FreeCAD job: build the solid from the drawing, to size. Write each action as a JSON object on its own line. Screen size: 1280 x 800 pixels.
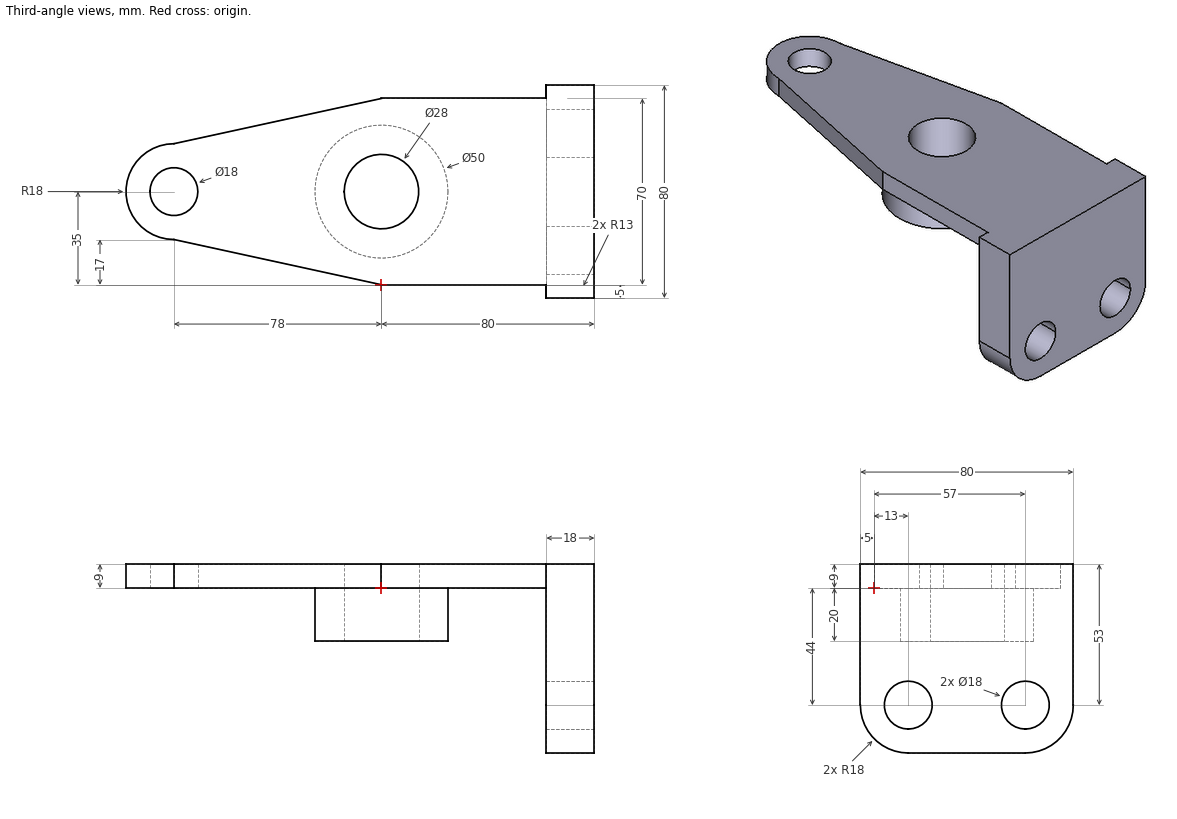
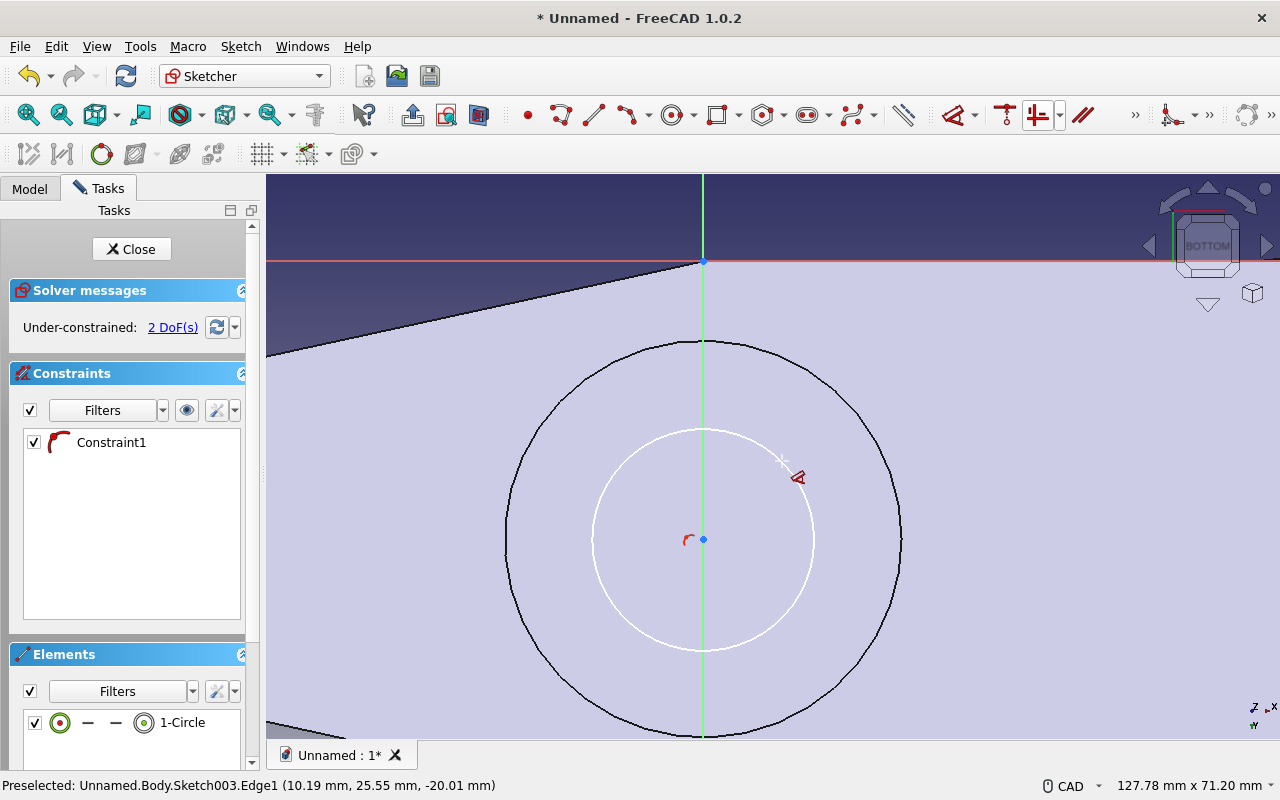
{"action": "left_click", "coordinate": [781, 461]}
{"action": "left_click", "coordinate": [803, 438]}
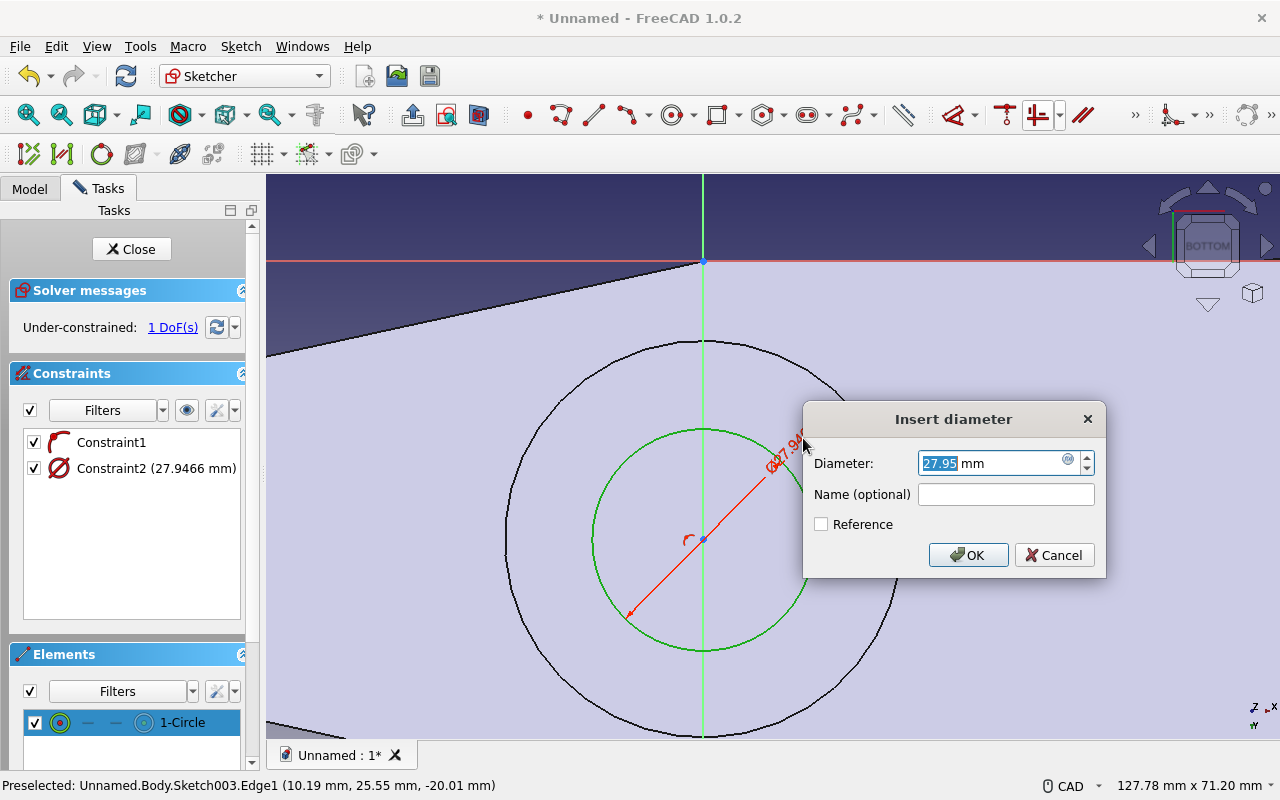
{"action": "type", "text": "28"}
{"action": "key", "text": "Return"}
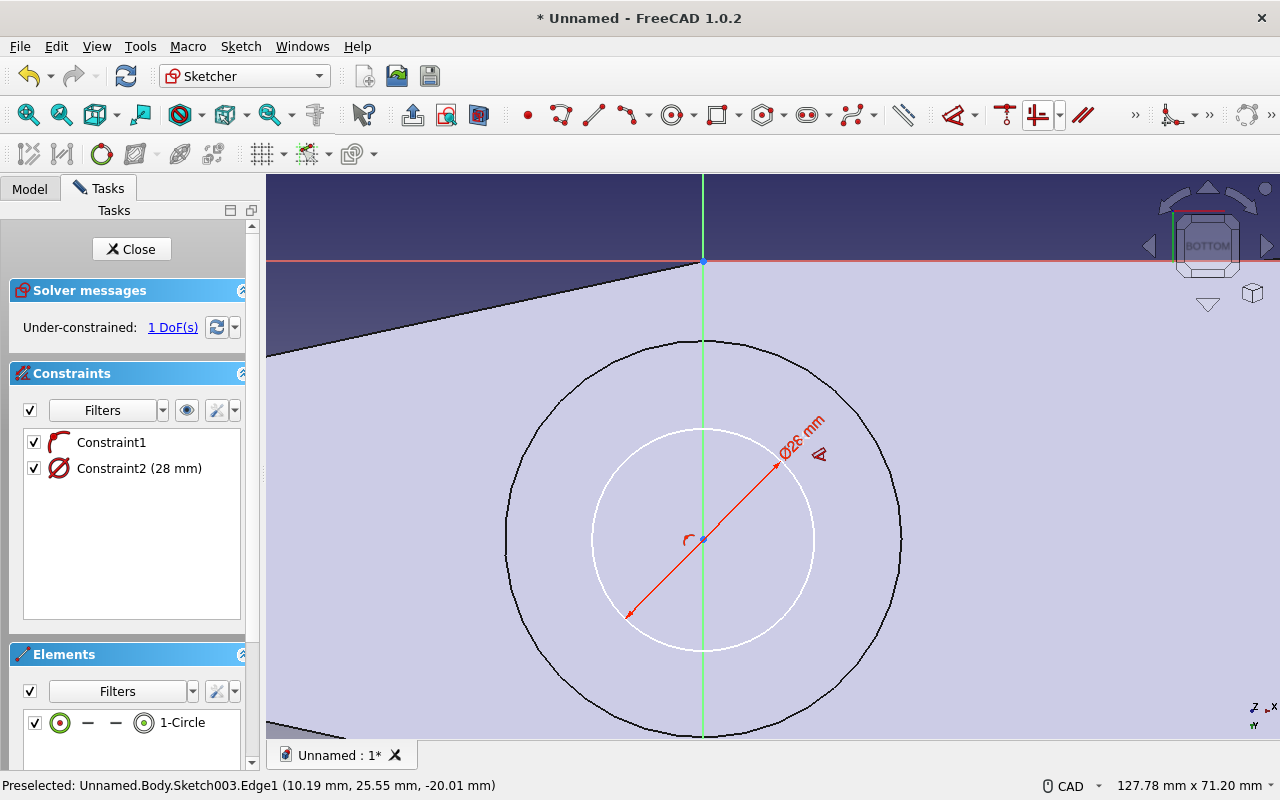
{"action": "left_click", "coordinate": [703, 540]}
{"action": "left_click", "coordinate": [737, 401]}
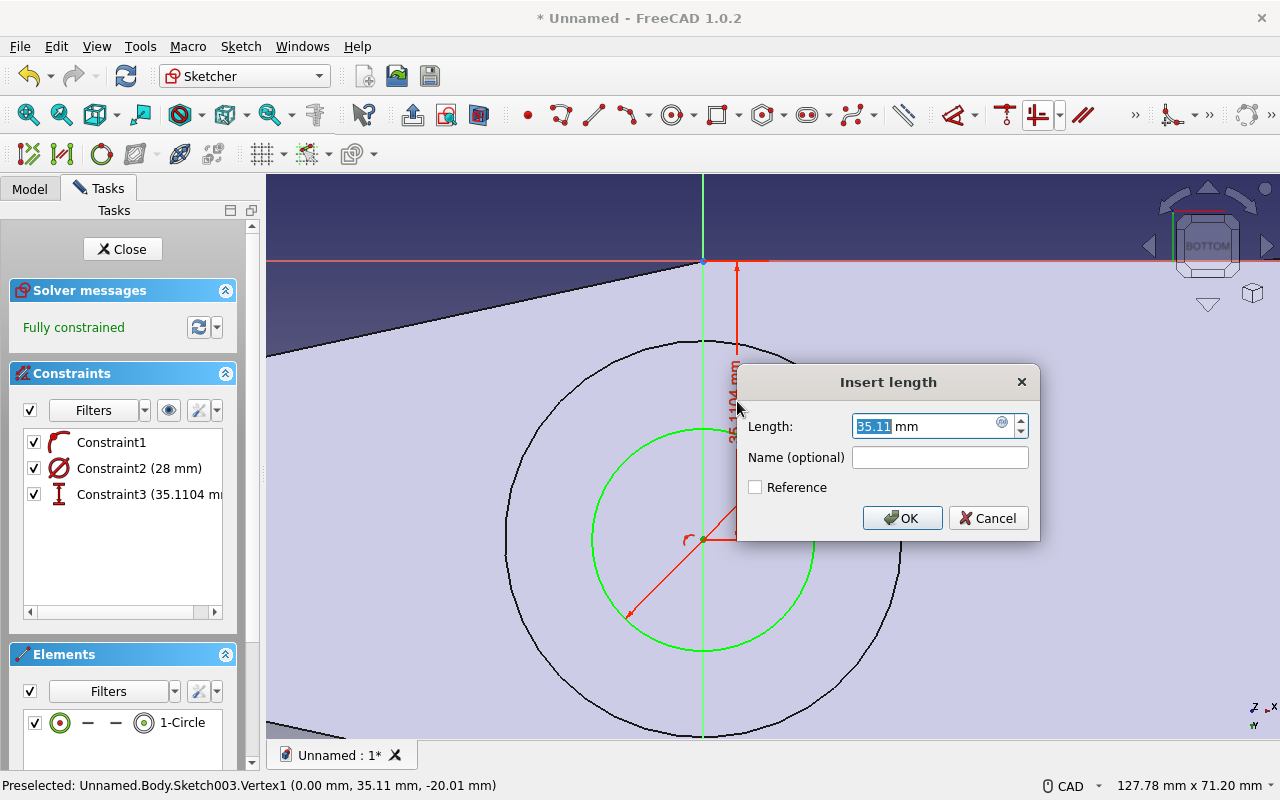
{"action": "type", "text": "35"}
{"action": "key", "text": "Return"}
{"action": "key", "text": "Escape"}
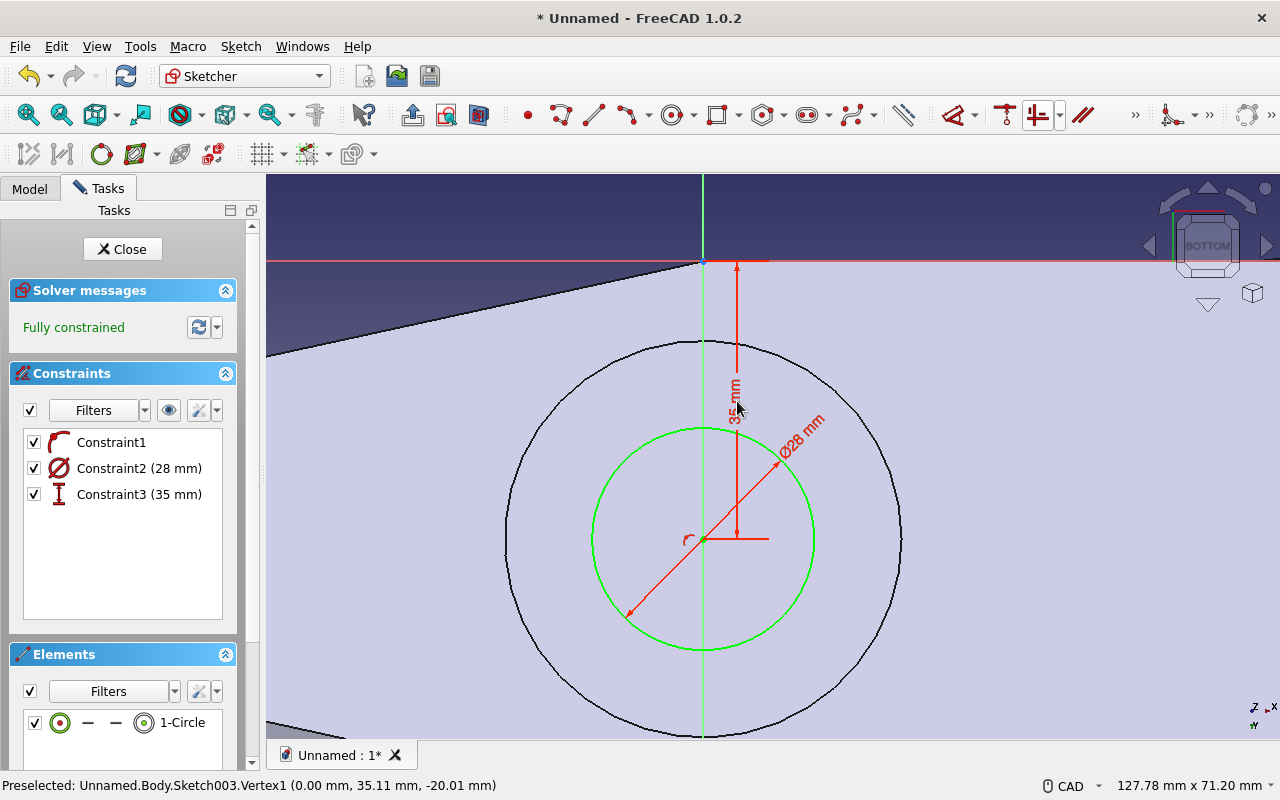
{"action": "left_click", "coordinate": [123, 249]}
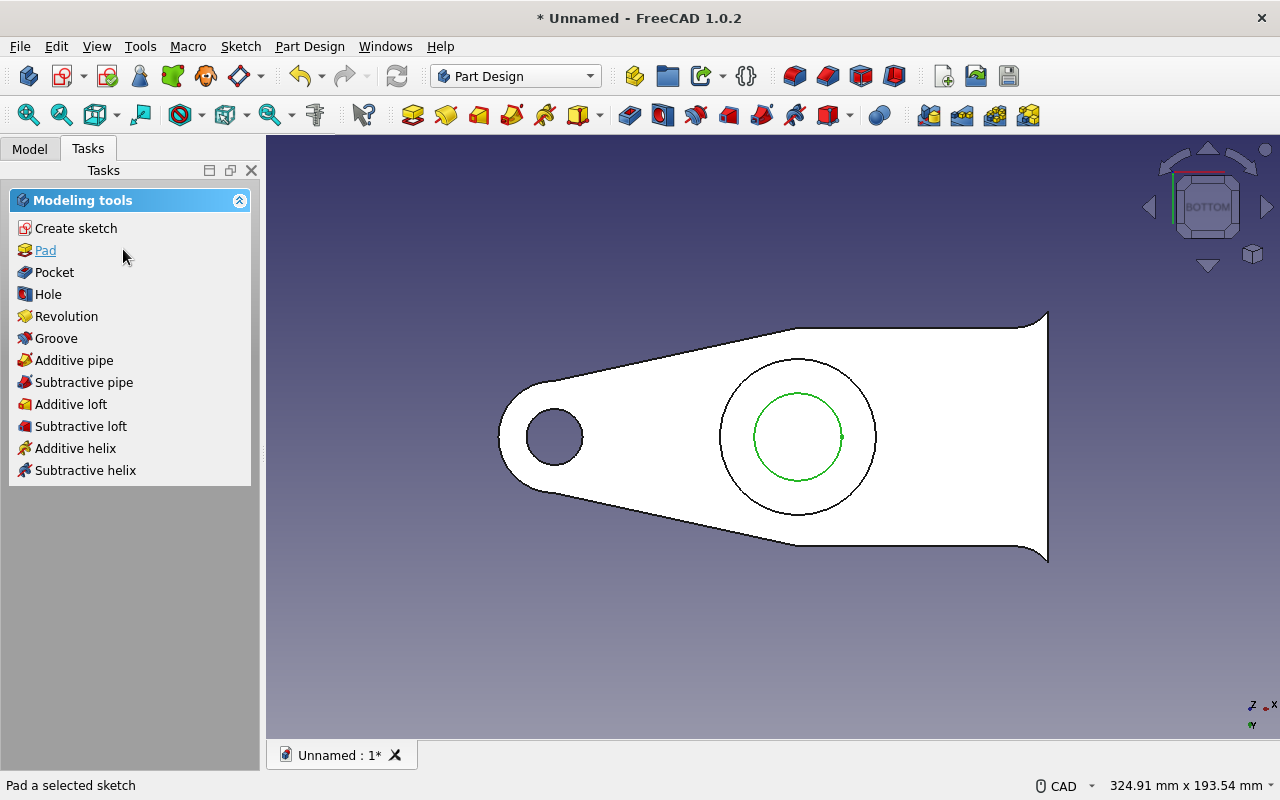
{"action": "left_click", "coordinate": [630, 116]}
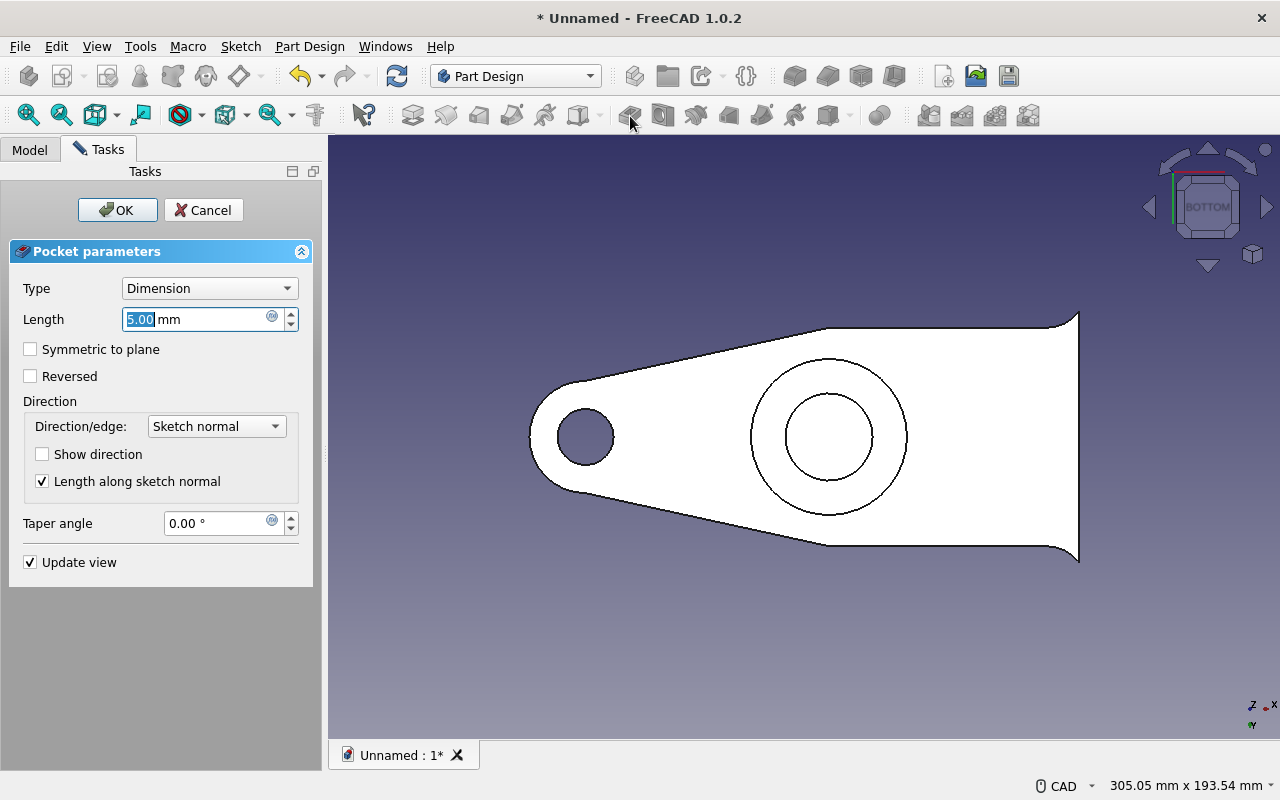
{"action": "left_click", "coordinate": [210, 288]}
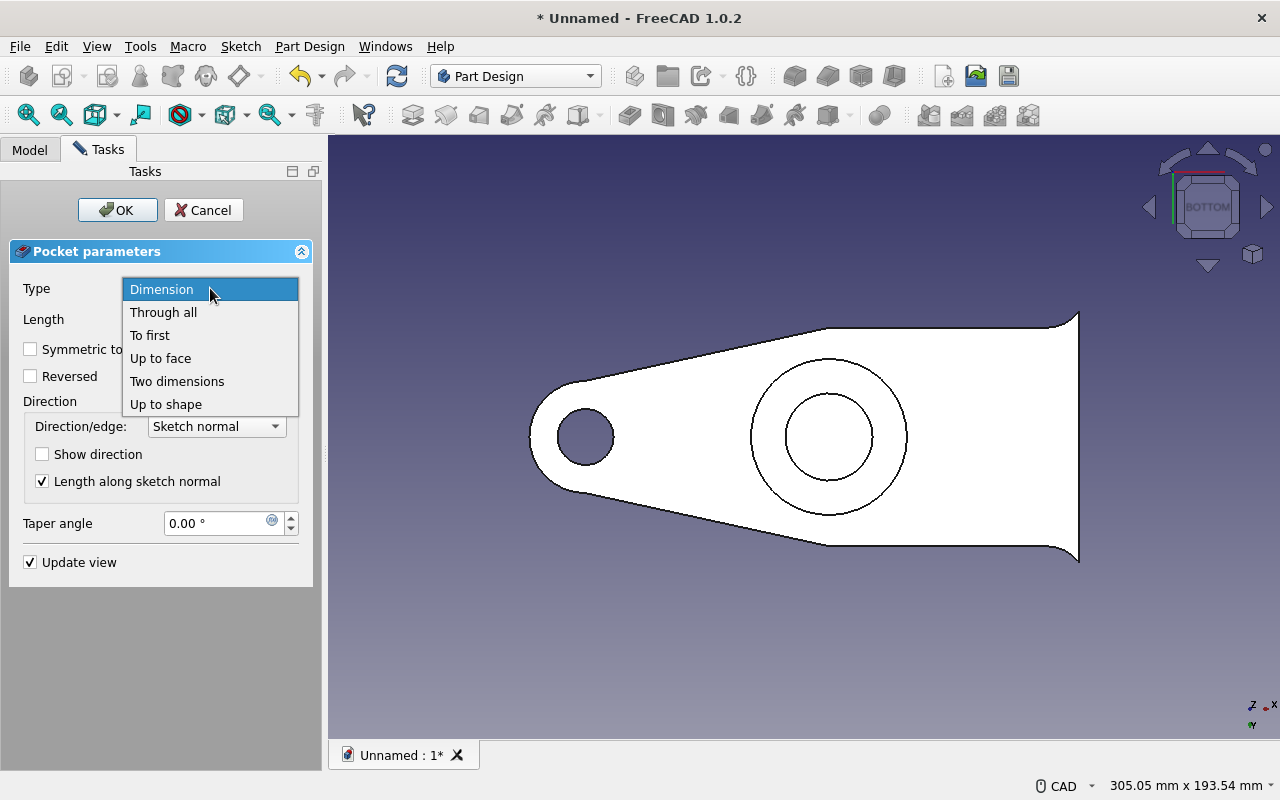
{"action": "left_click", "coordinate": [208, 312]}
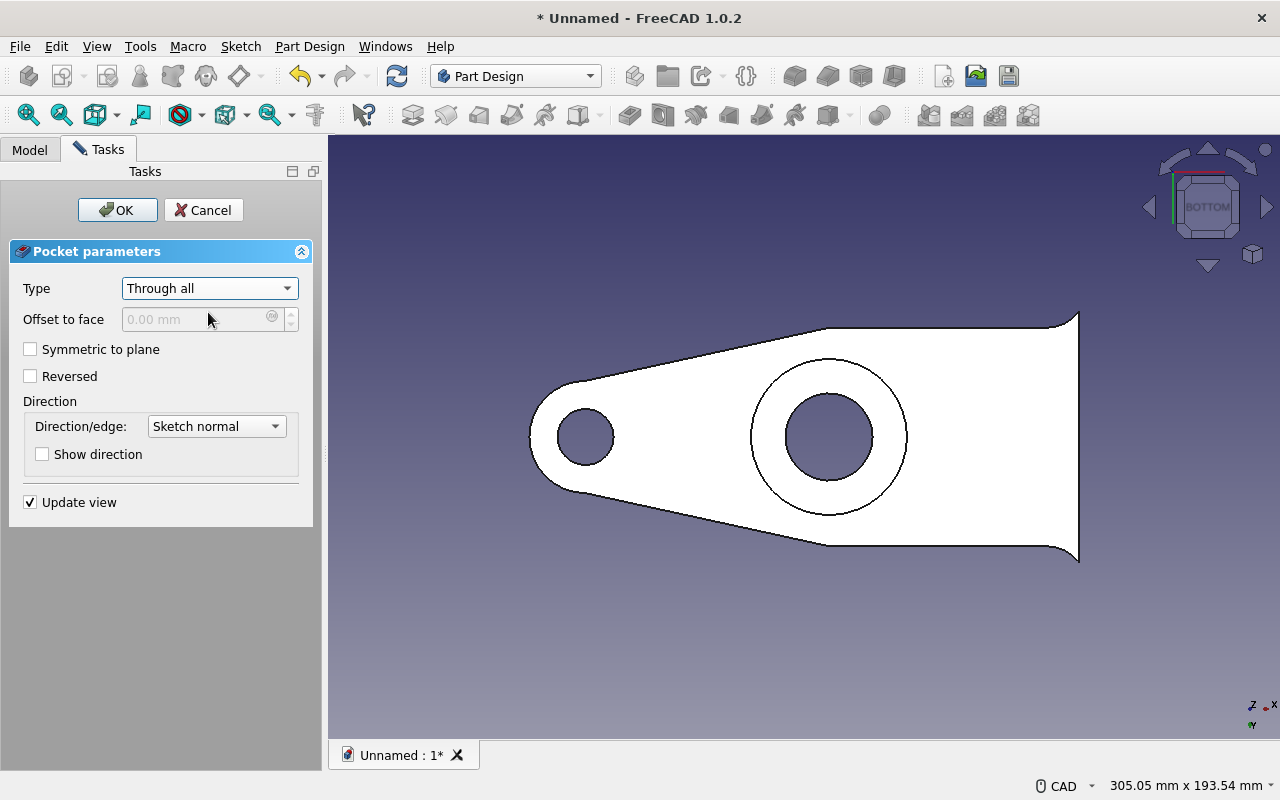
{"action": "left_click", "coordinate": [118, 210]}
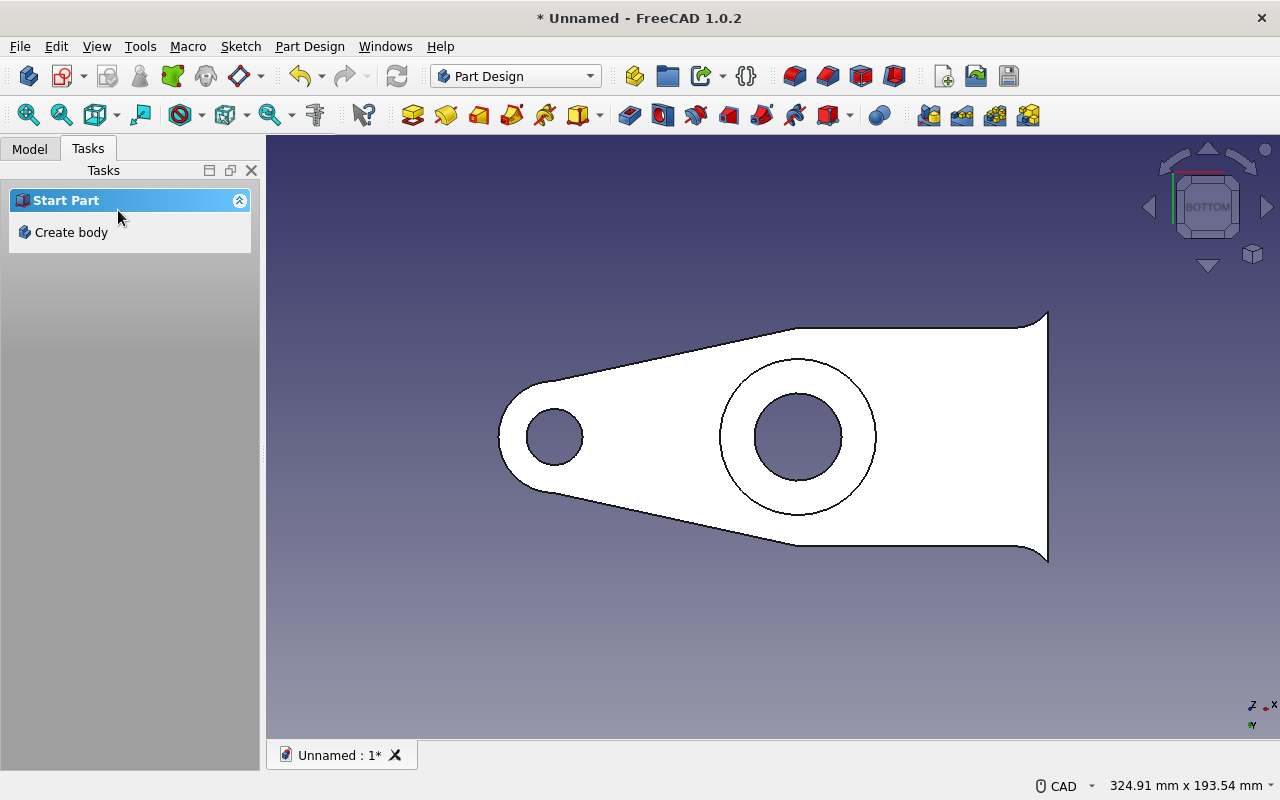
{"action": "key", "text": "0"}